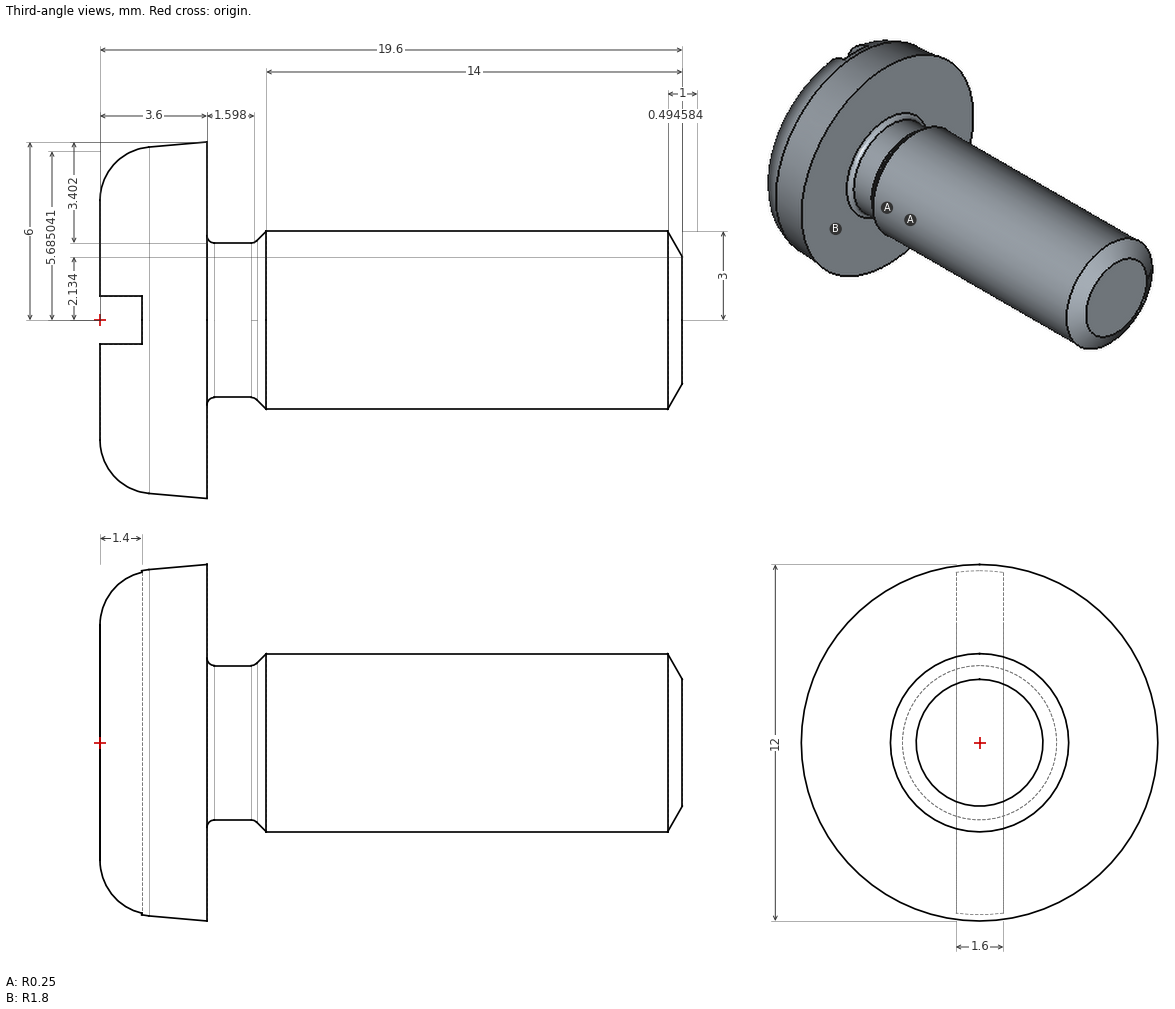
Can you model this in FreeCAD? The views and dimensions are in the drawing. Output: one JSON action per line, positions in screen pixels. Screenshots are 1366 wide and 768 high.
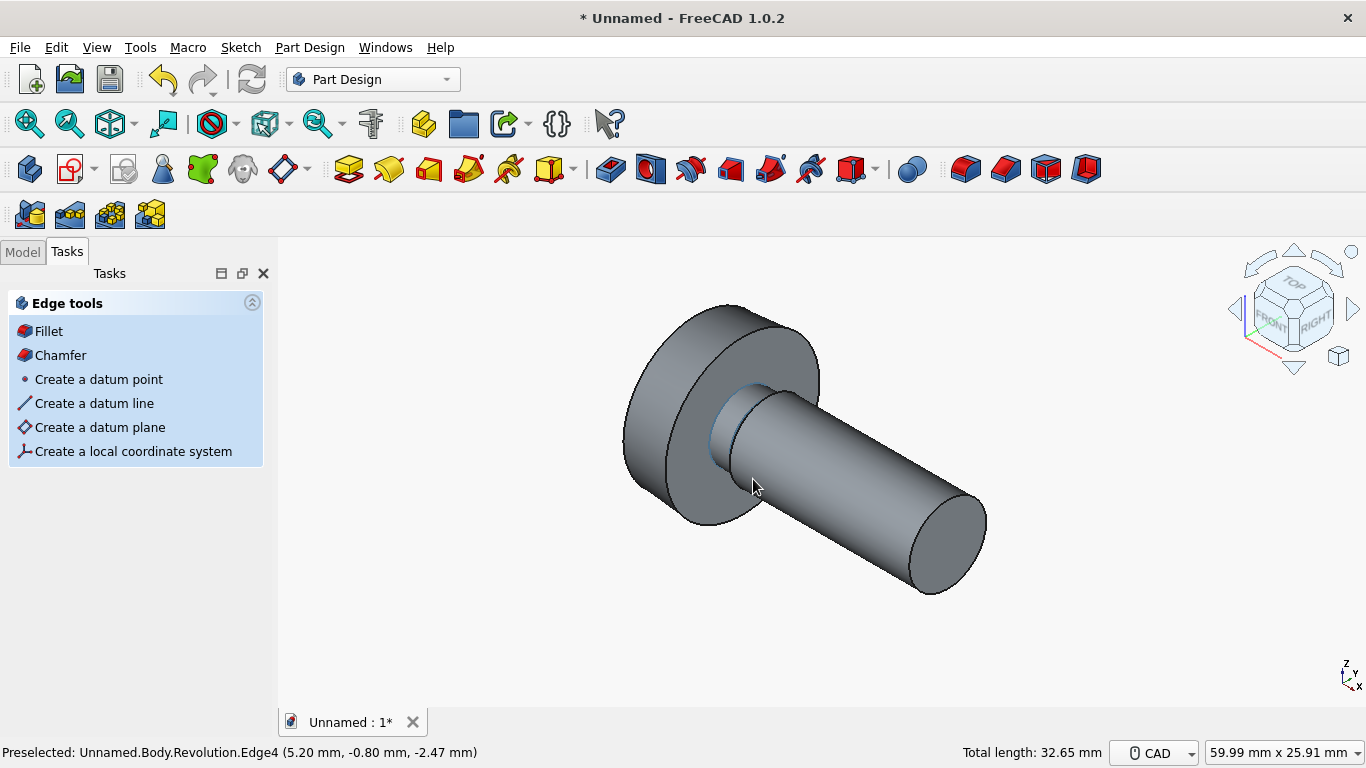
{"action": "left_click", "coordinate": [966, 170]}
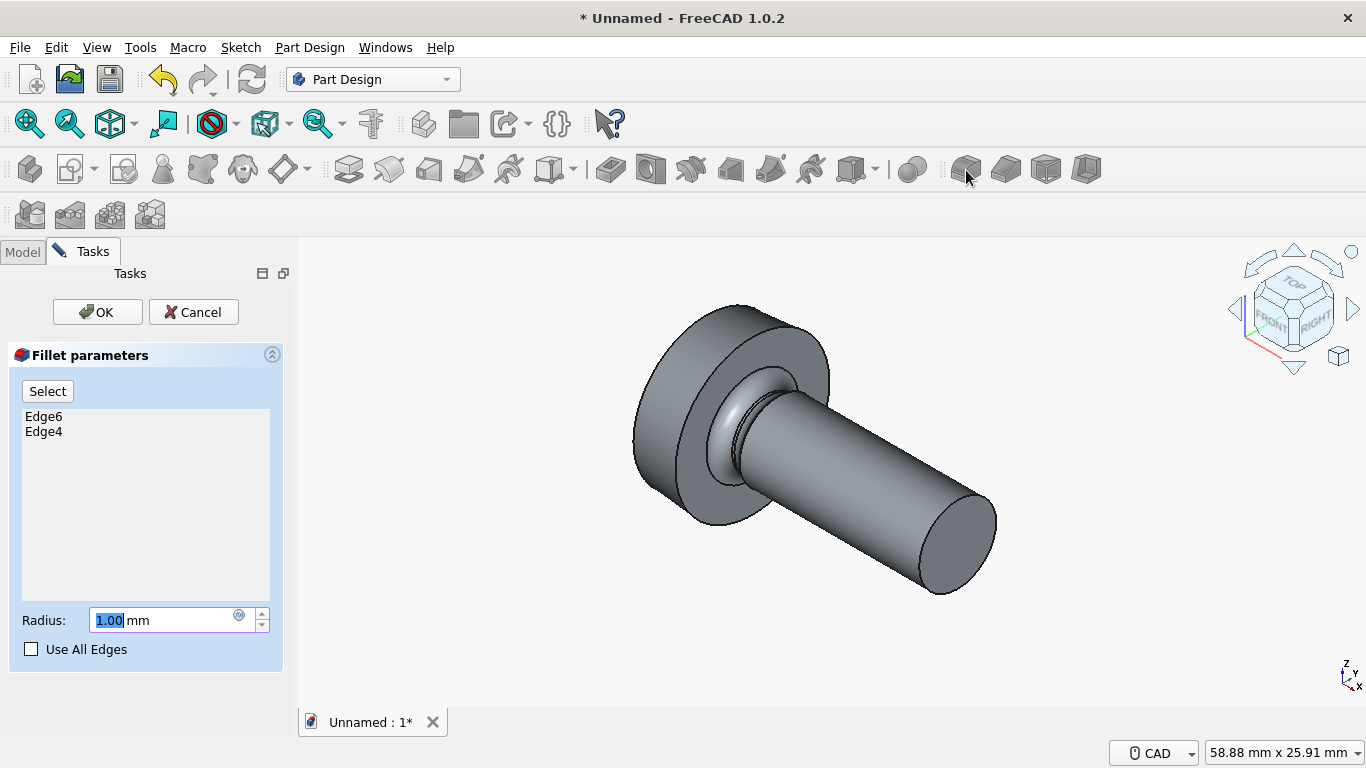
{"action": "type", "text": "0.25"}
{"action": "key", "text": "Tab"}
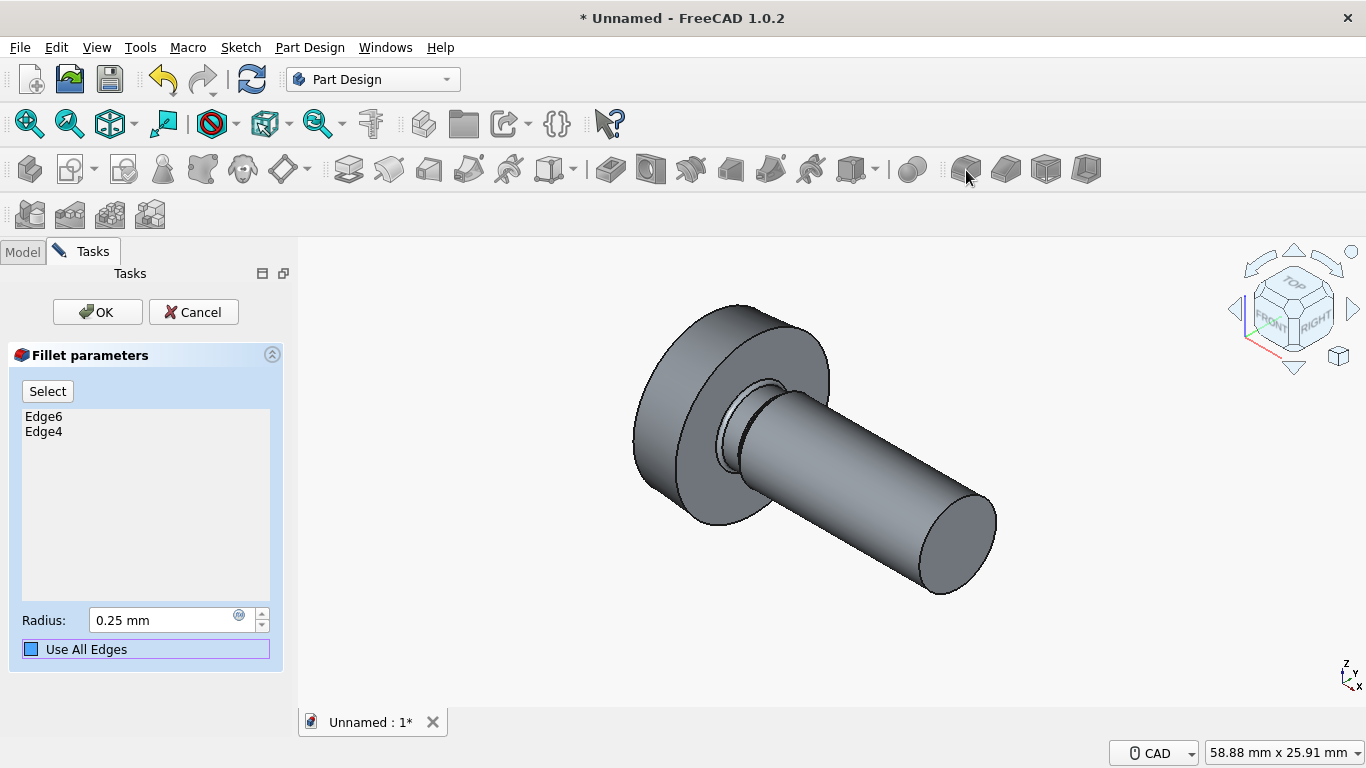
{"action": "left_click", "coordinate": [98, 312]}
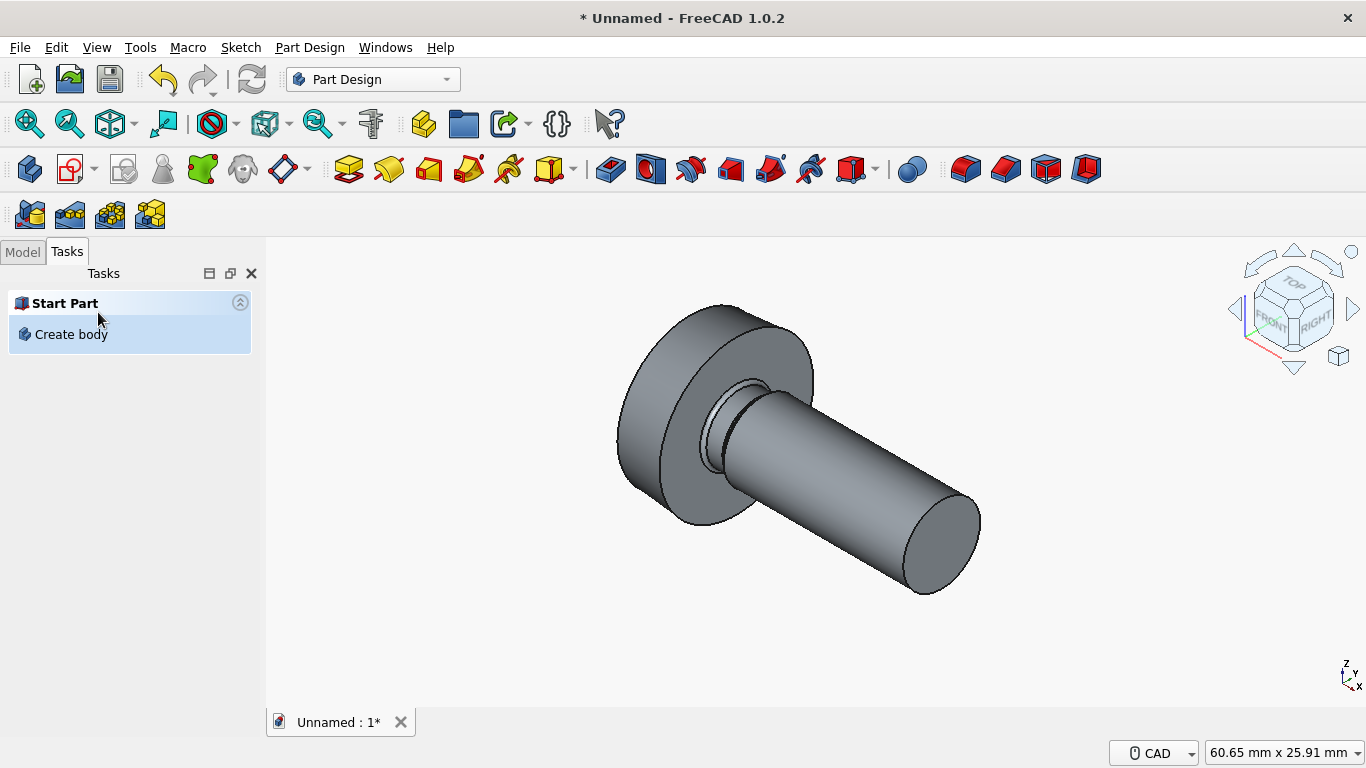
{"action": "left_click", "coordinate": [713, 305]}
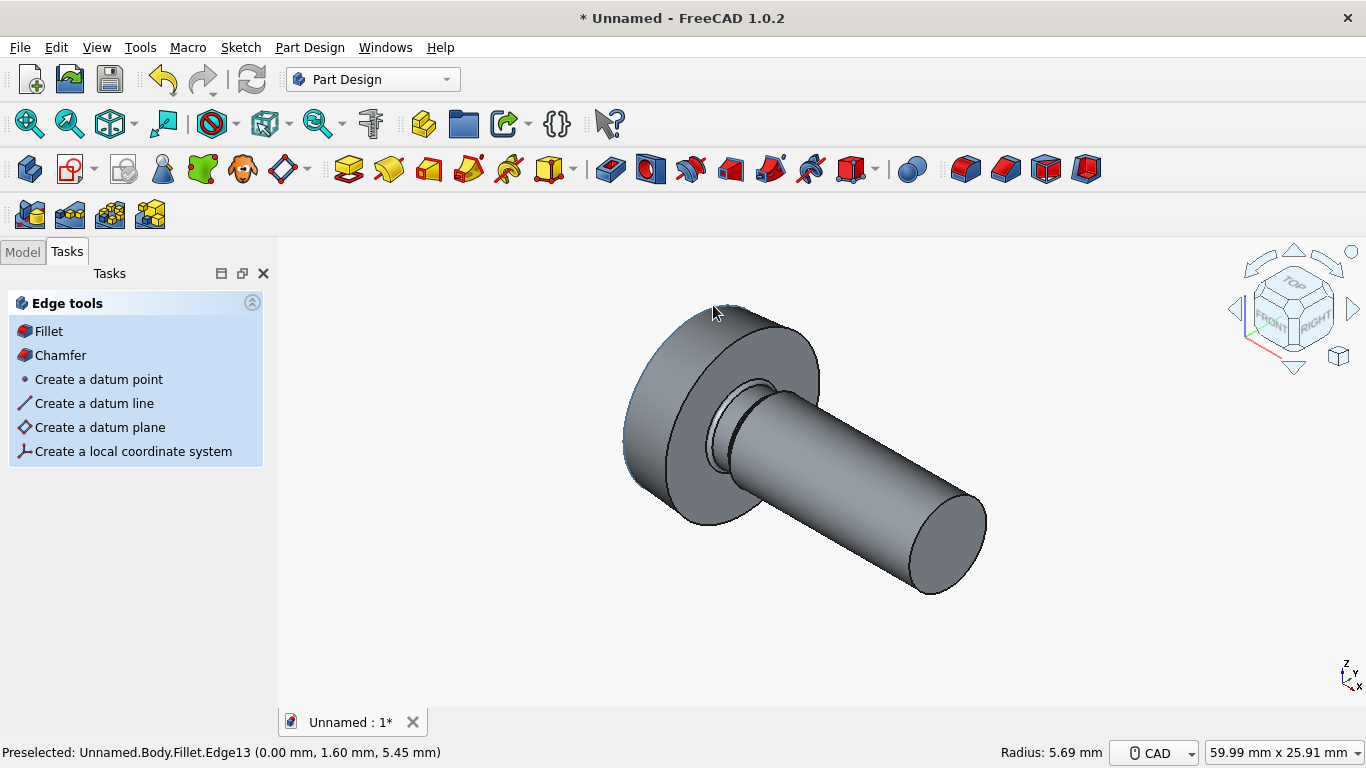
{"action": "left_click", "coordinate": [966, 170]}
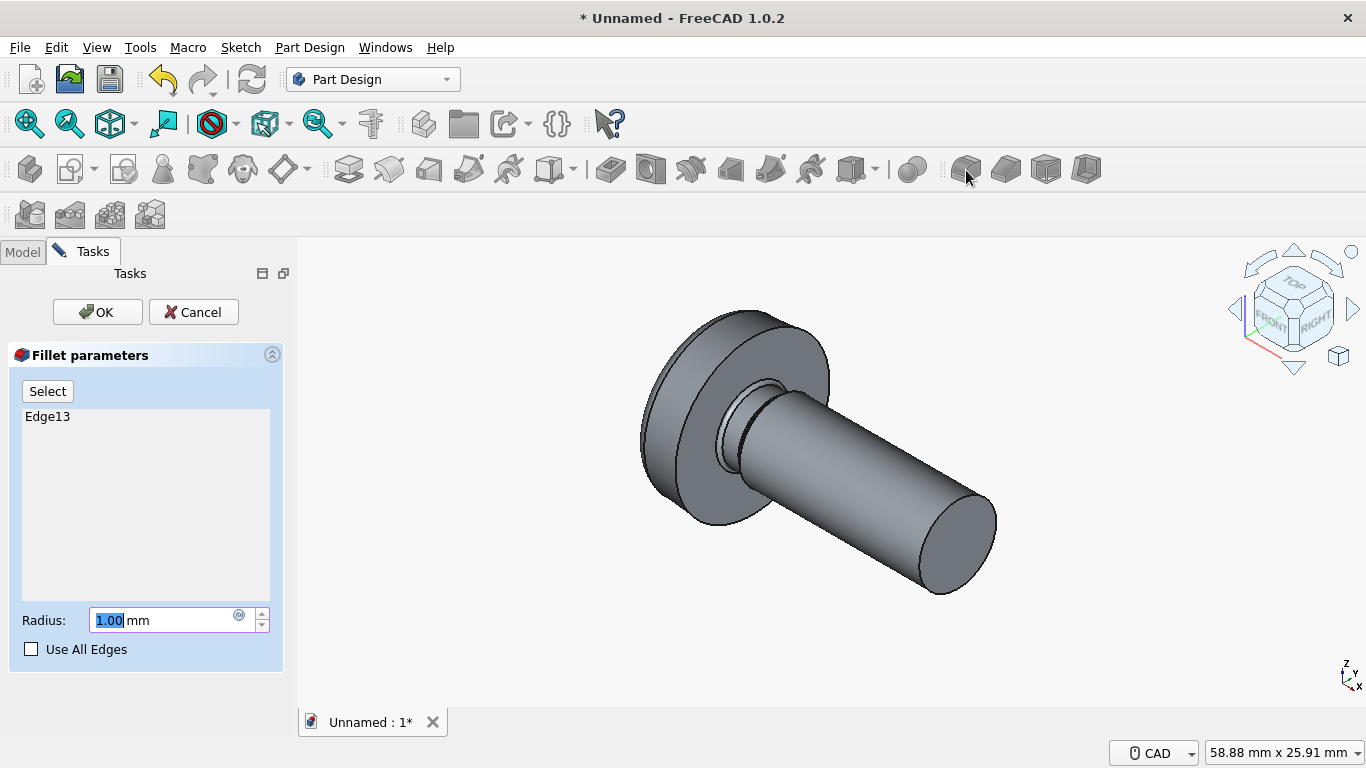
{"action": "type", "text": "1.8"}
{"action": "key", "text": "Tab"}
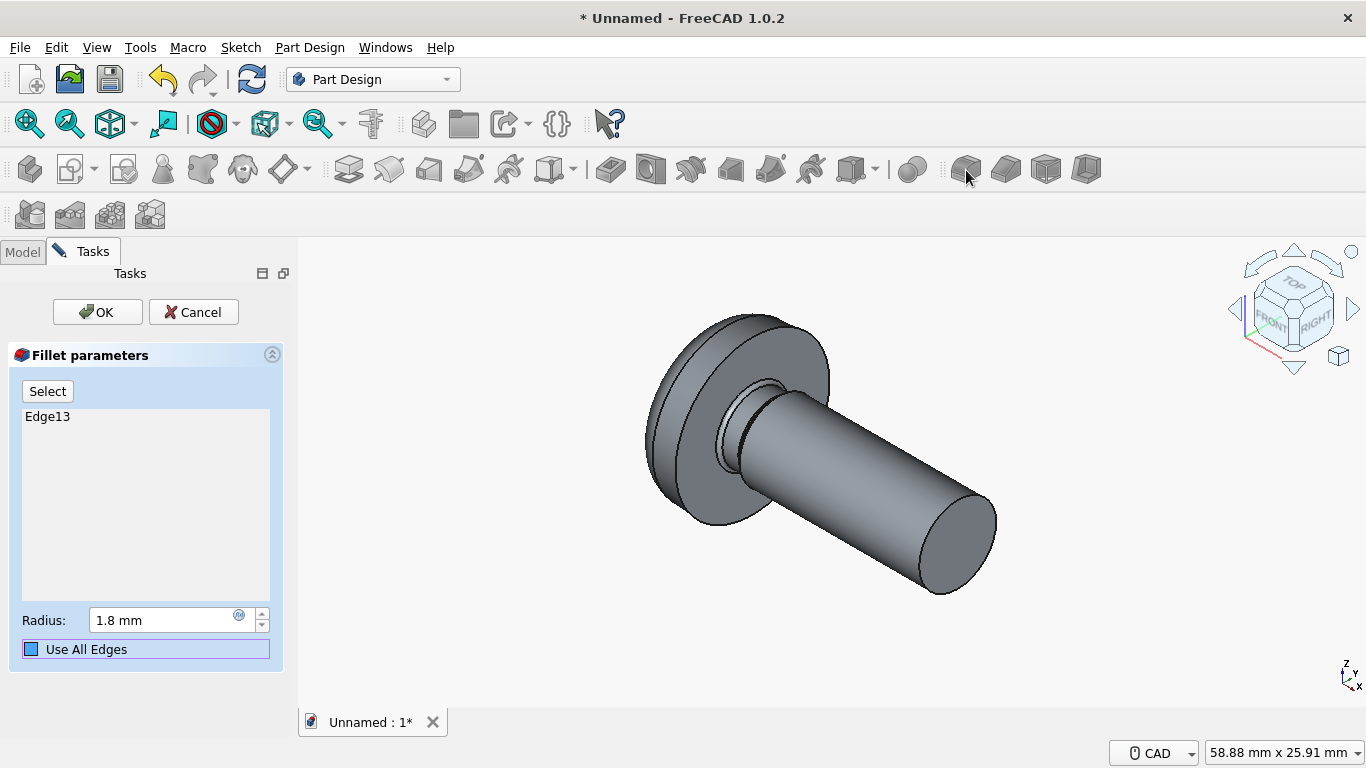
{"action": "left_click", "coordinate": [98, 312]}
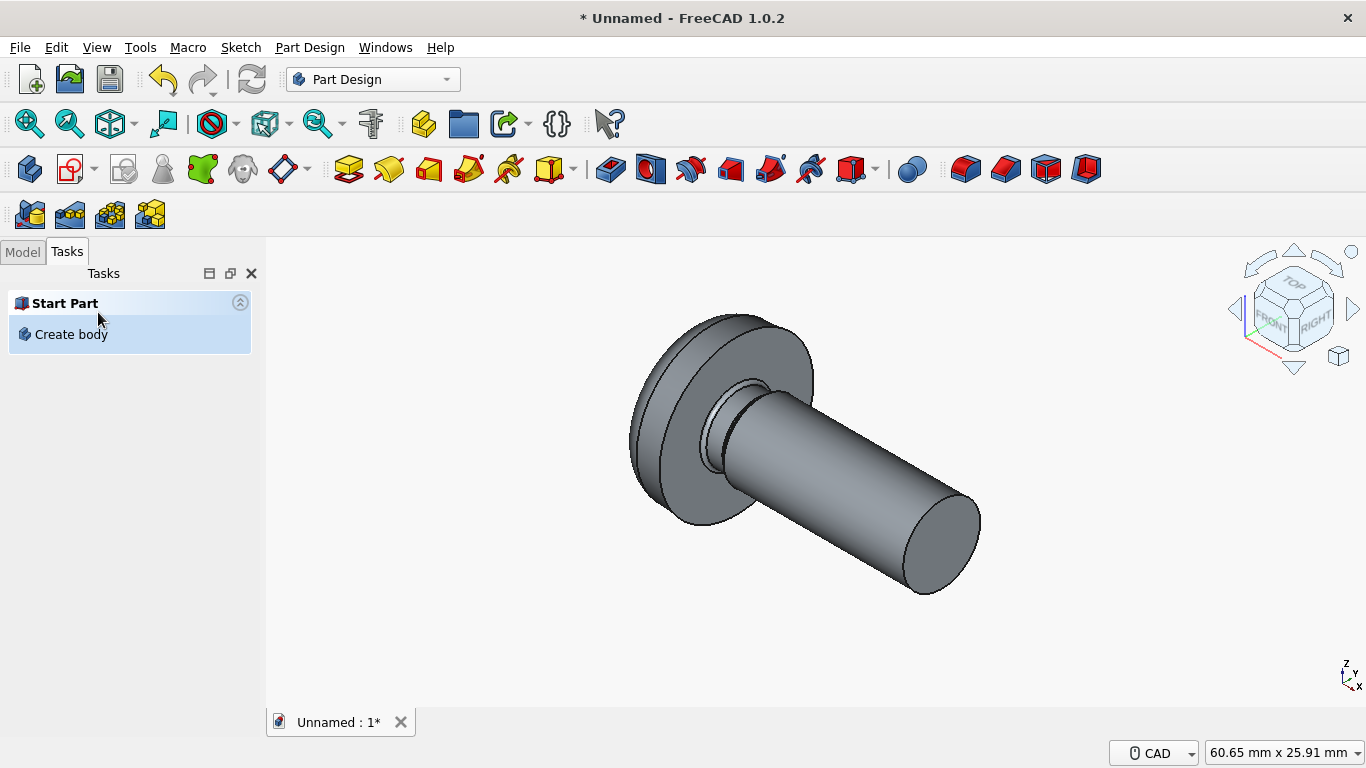
{"action": "key", "text": "6"}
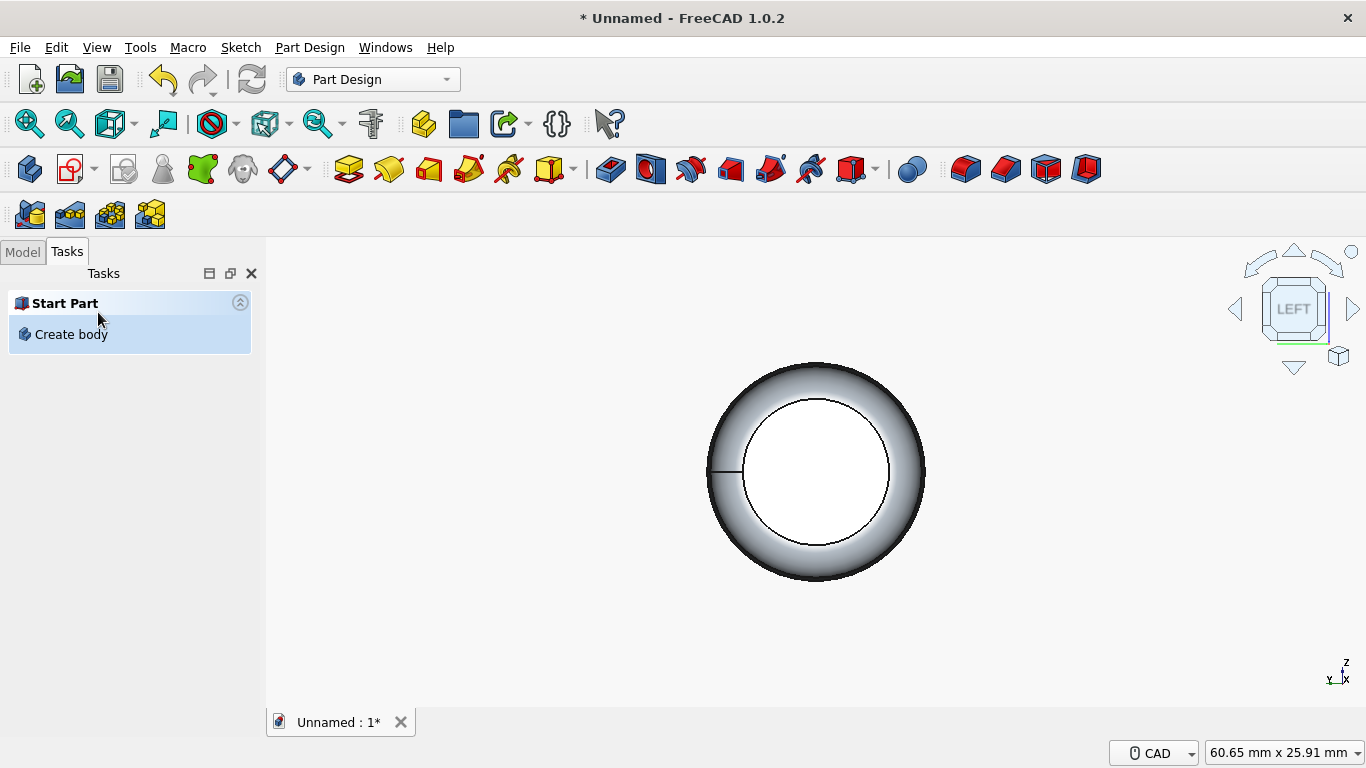
{"action": "left_click", "coordinate": [816, 471]}